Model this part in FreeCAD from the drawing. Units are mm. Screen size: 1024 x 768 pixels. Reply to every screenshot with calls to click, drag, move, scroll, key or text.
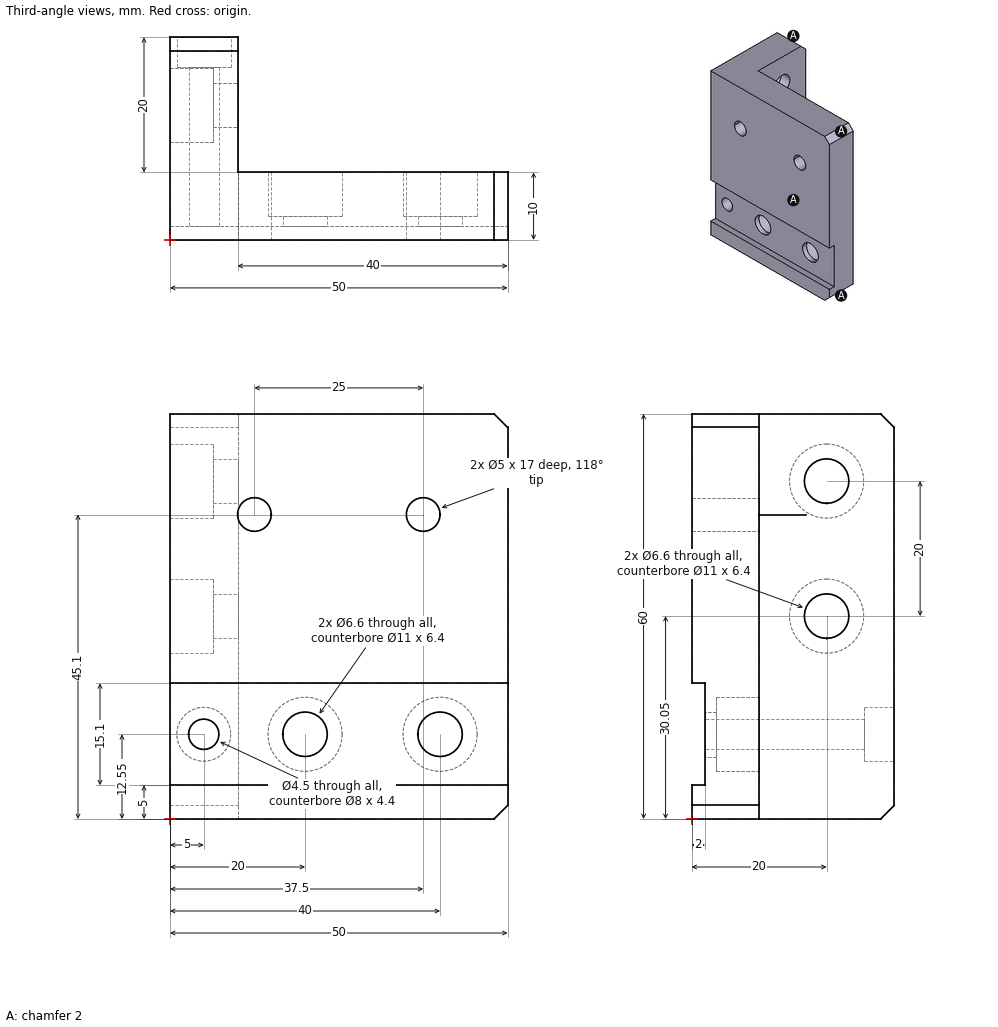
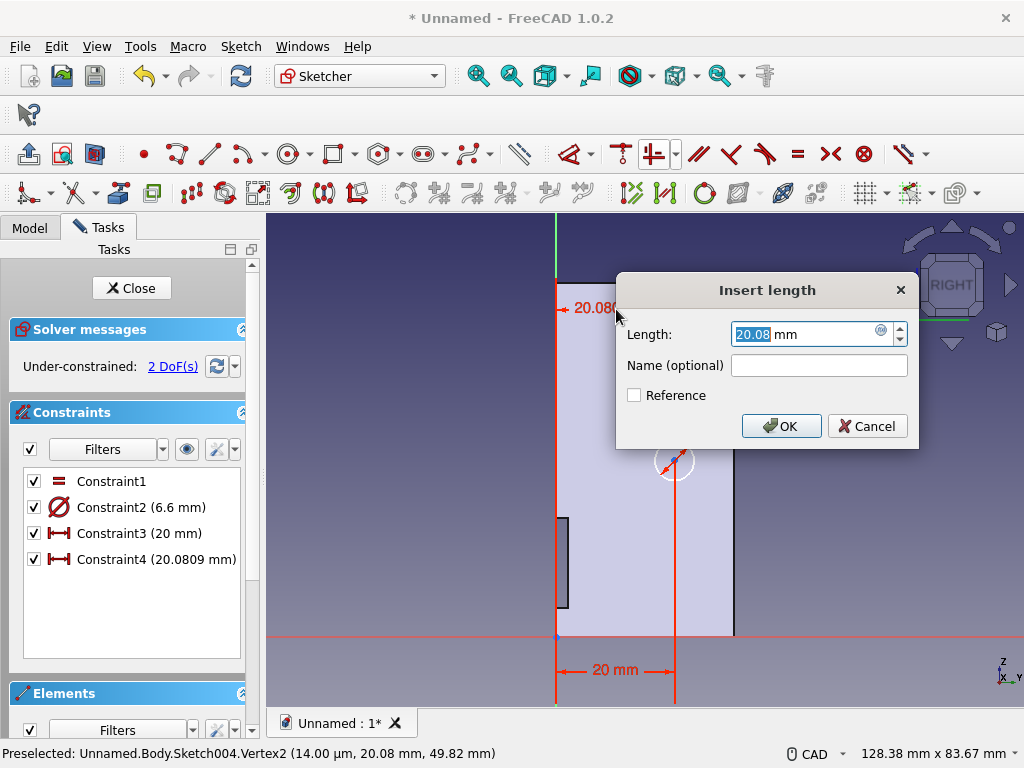
text(20)
key(Return)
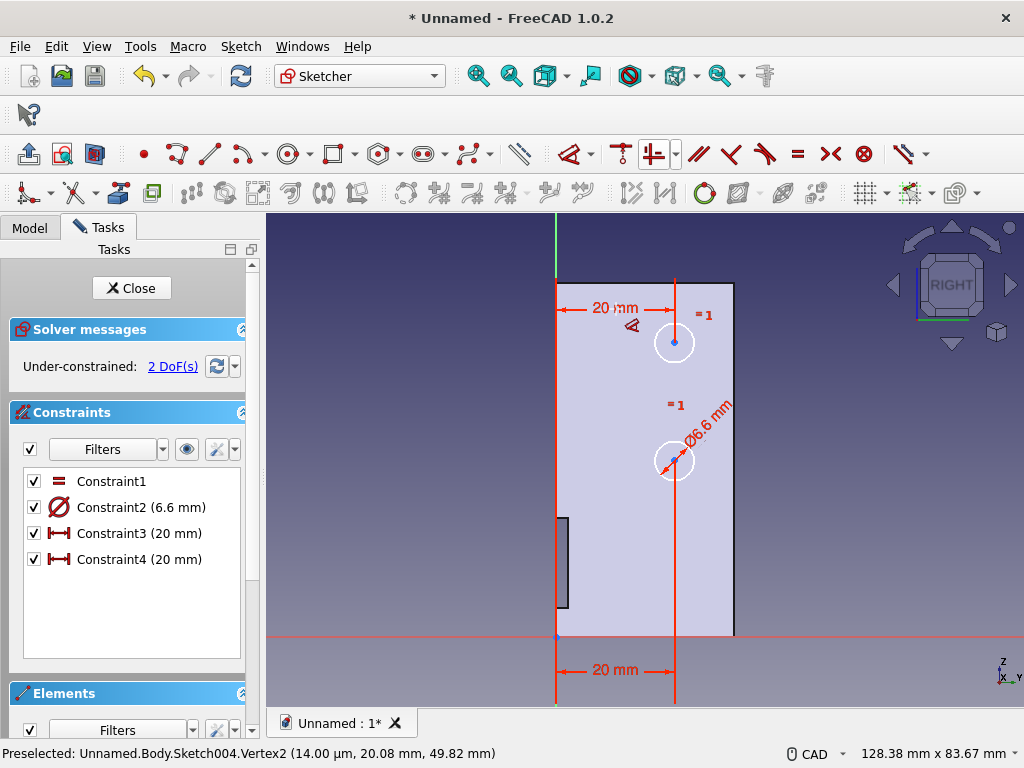
click(675, 461)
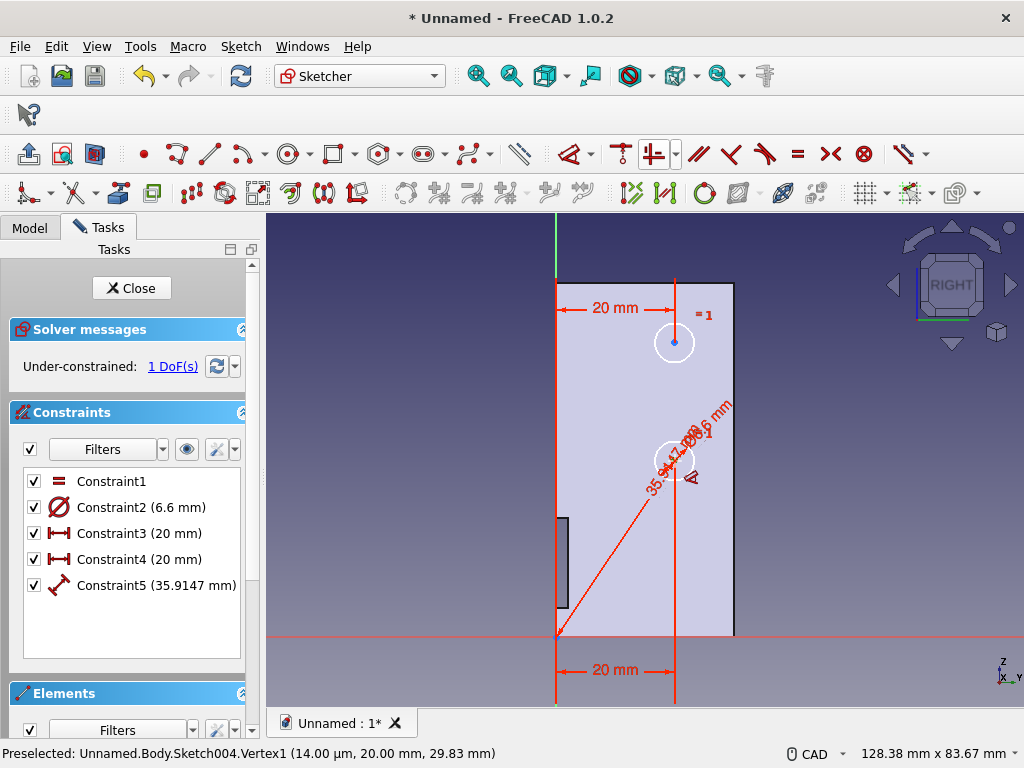
click(675, 343)
click(709, 402)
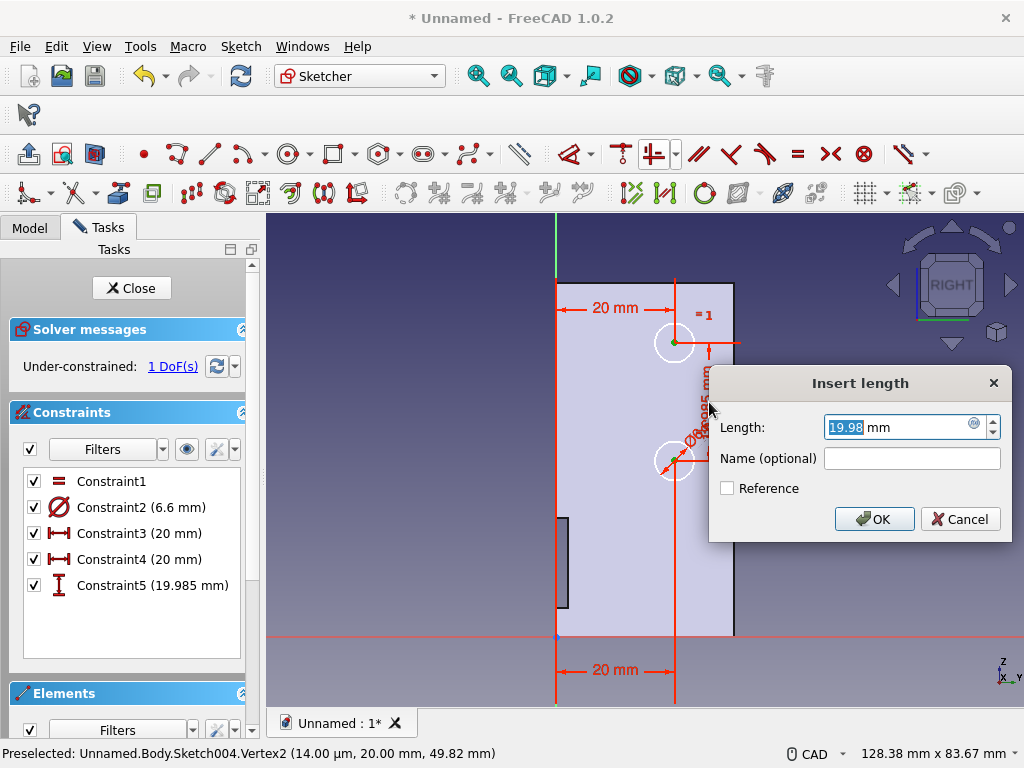
text(20)
key(Return)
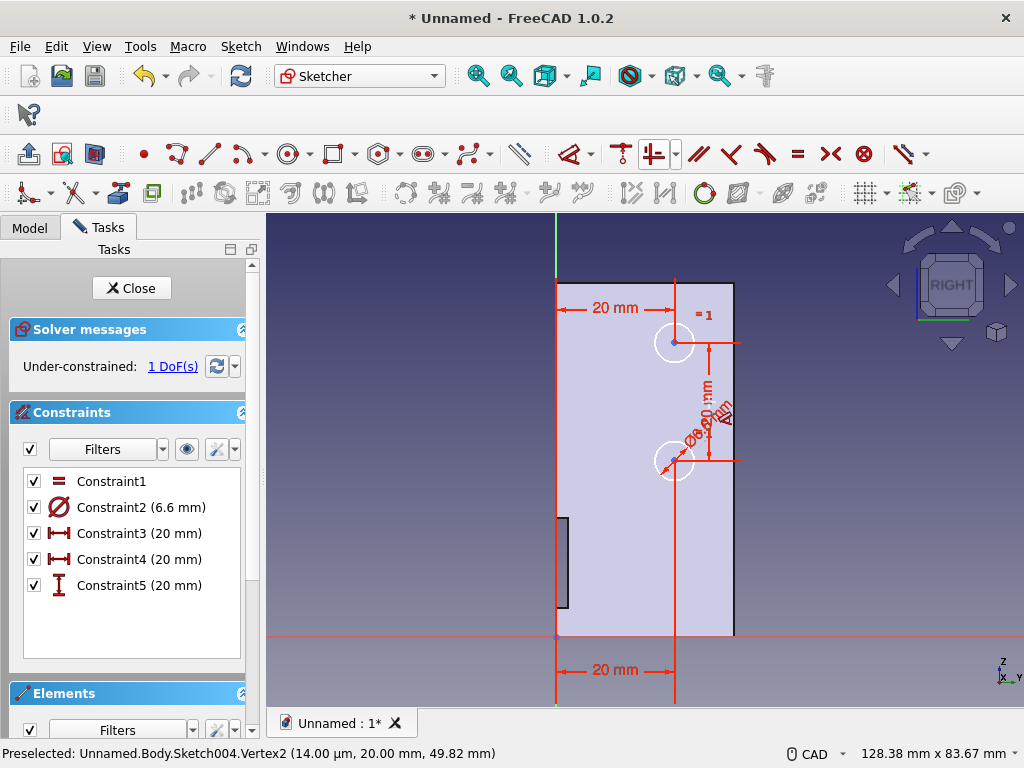
click(675, 461)
click(522, 549)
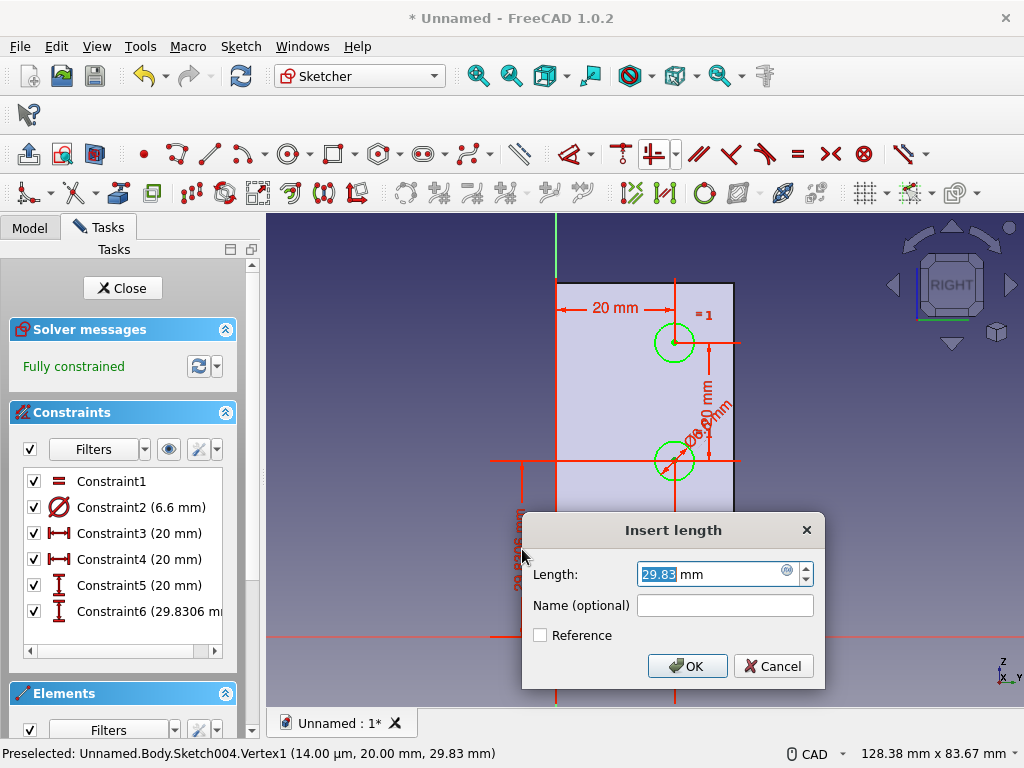
text(30.05)
key(Return)
key(Escape)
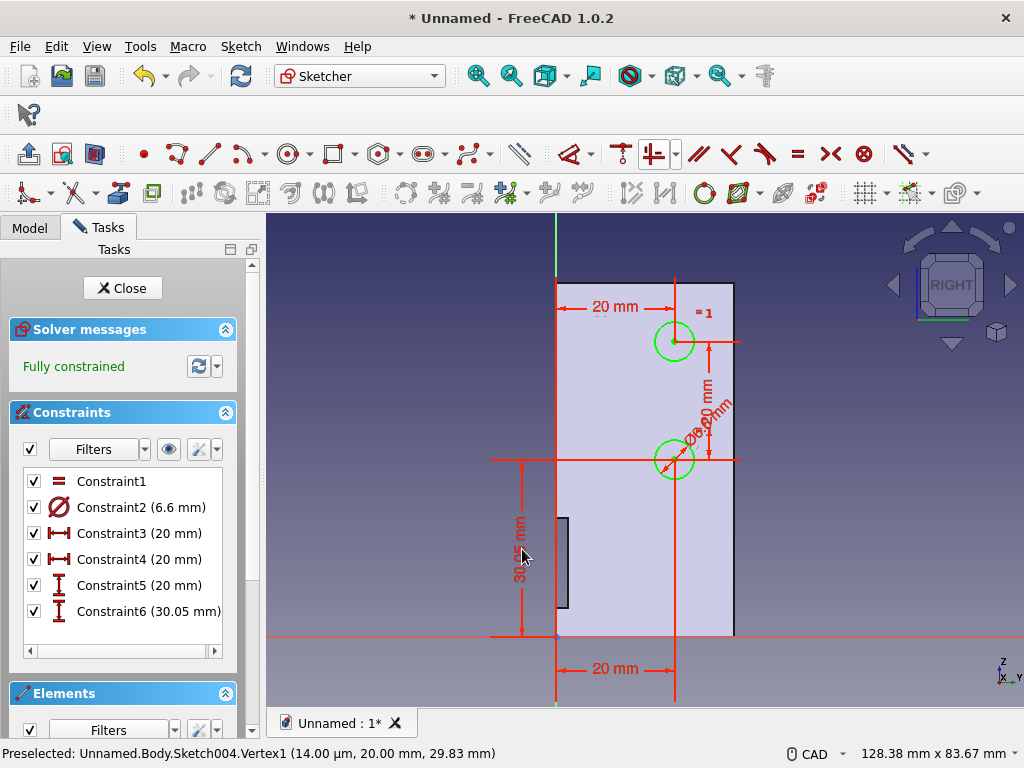
click(123, 288)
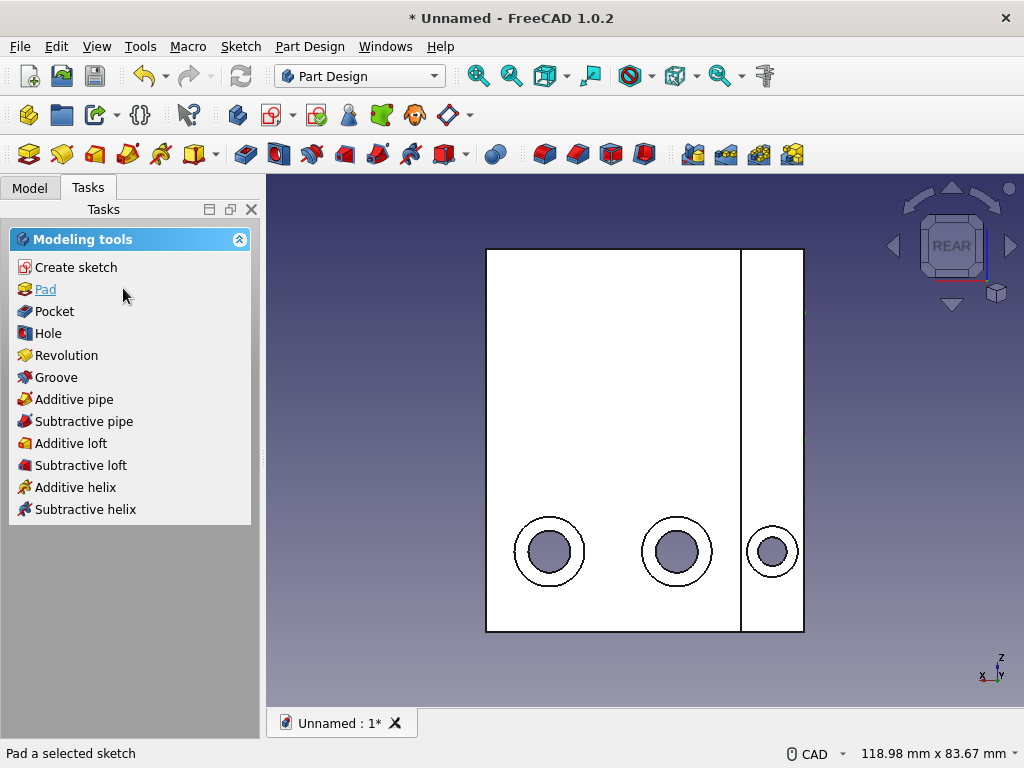
click(279, 154)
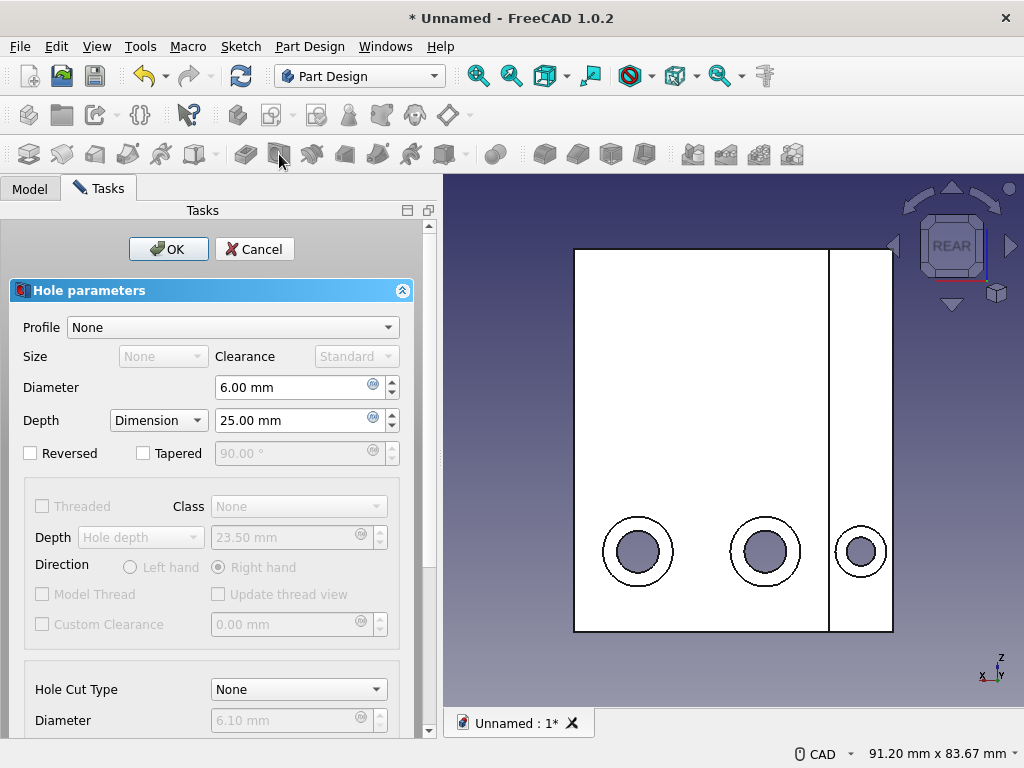
triple_click(300, 388)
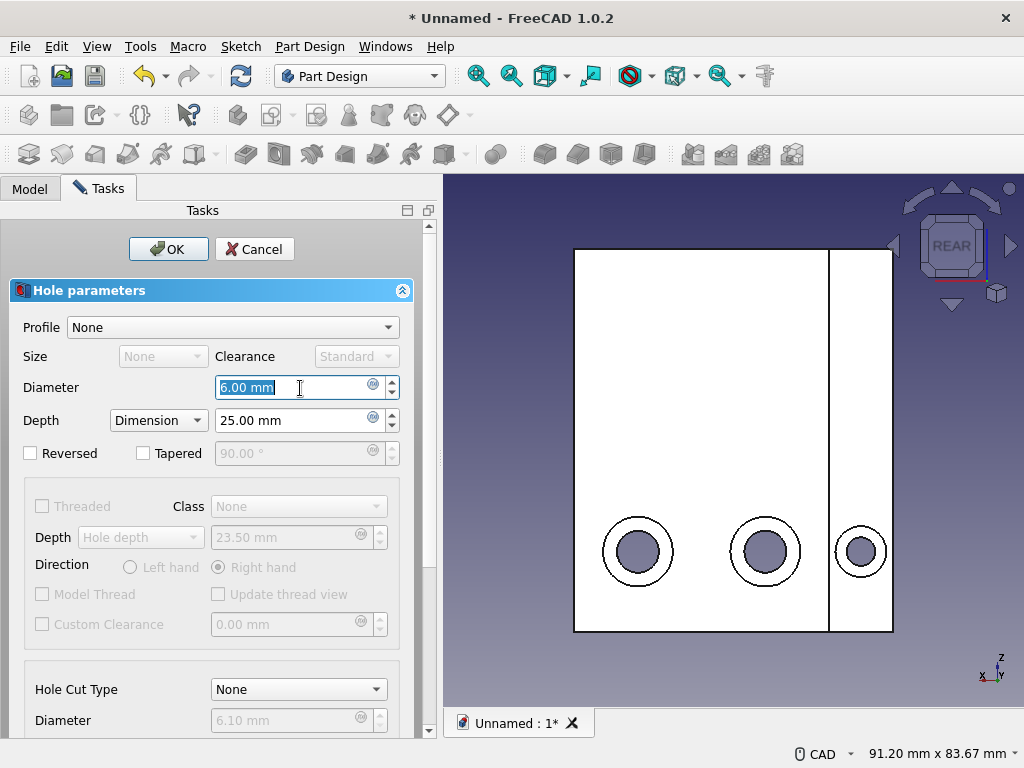
text(6.6)
key(Tab)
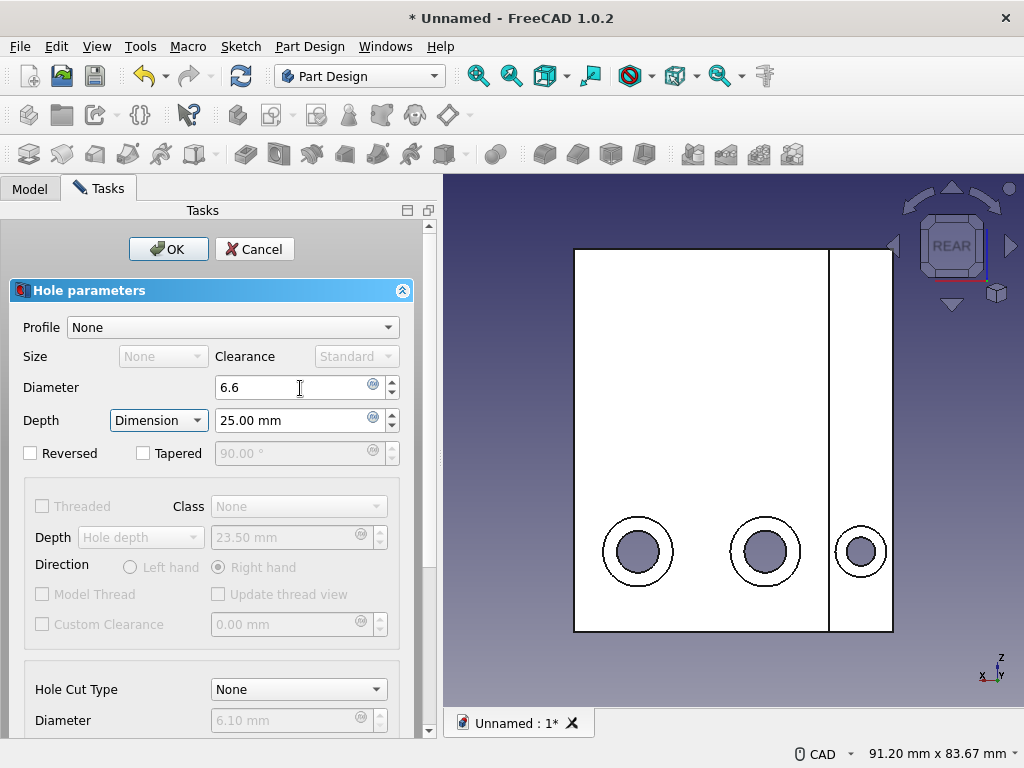
click(160, 420)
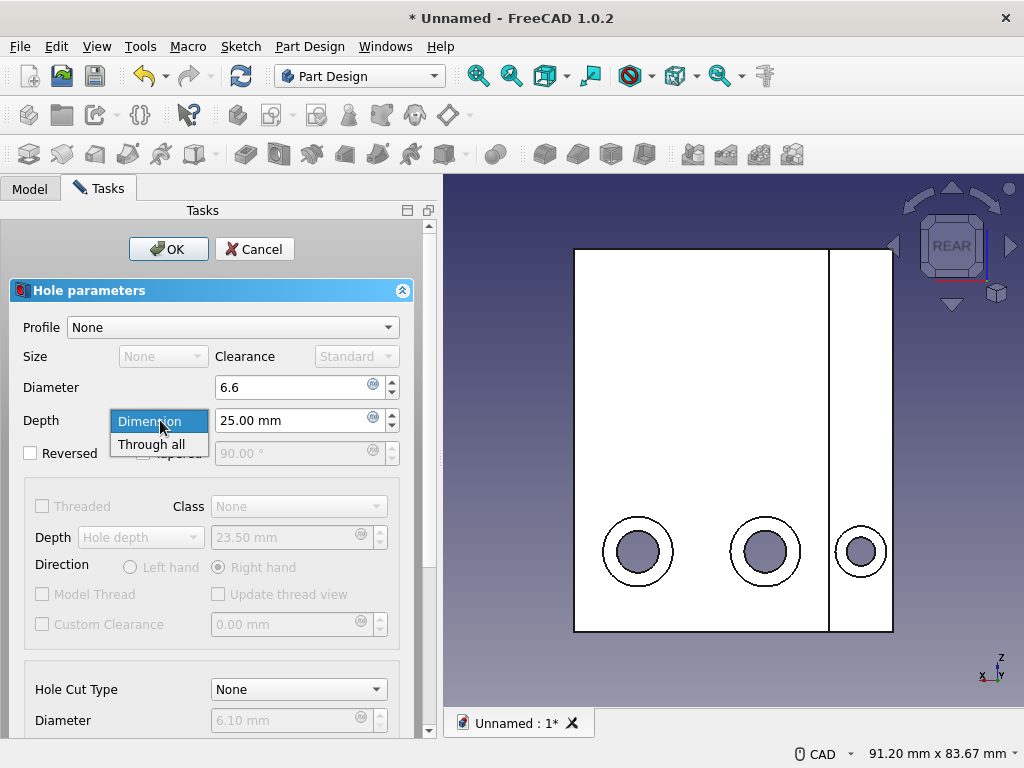
click(158, 444)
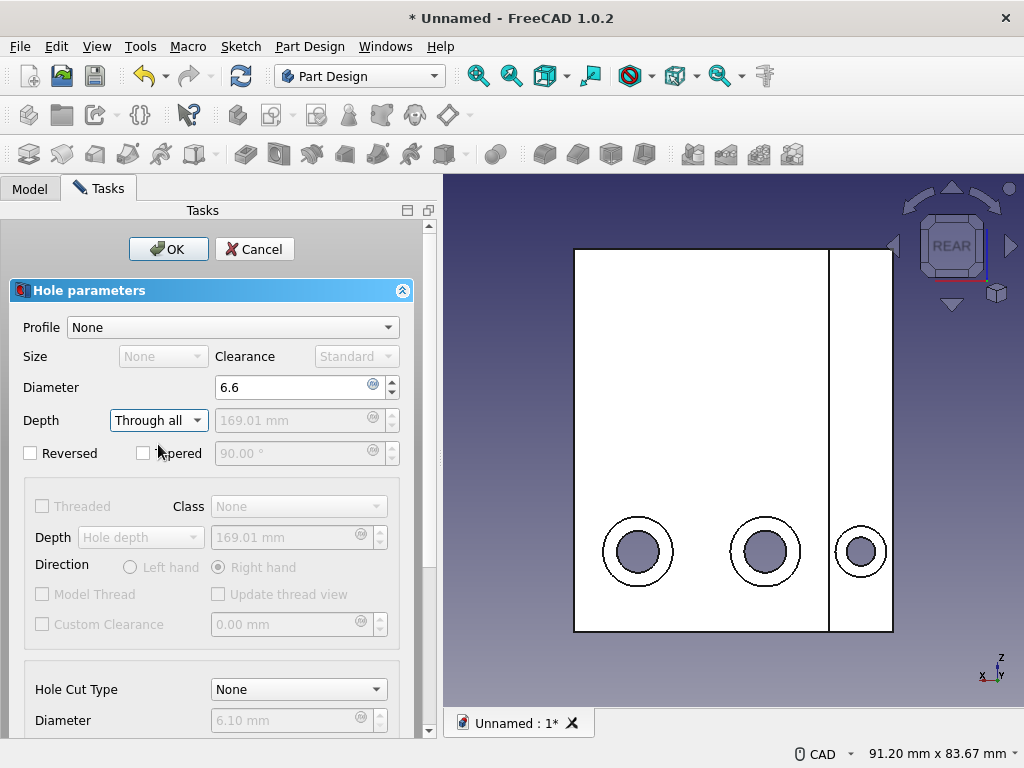
click(31, 453)